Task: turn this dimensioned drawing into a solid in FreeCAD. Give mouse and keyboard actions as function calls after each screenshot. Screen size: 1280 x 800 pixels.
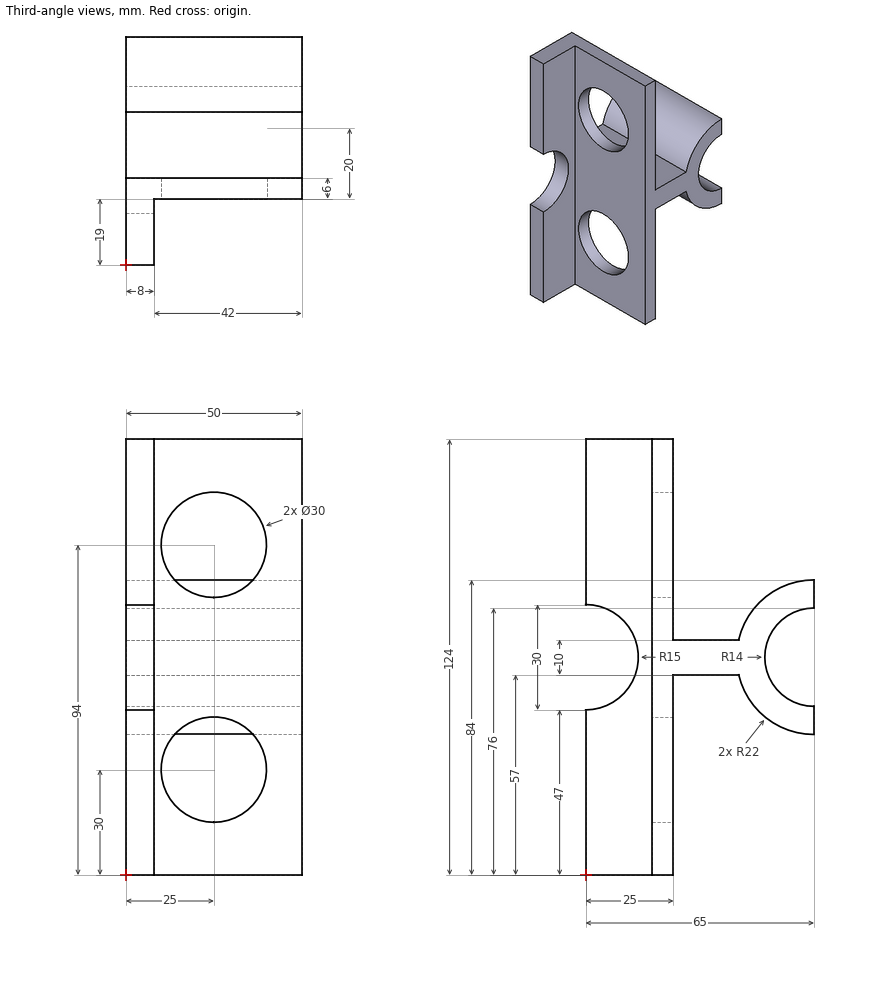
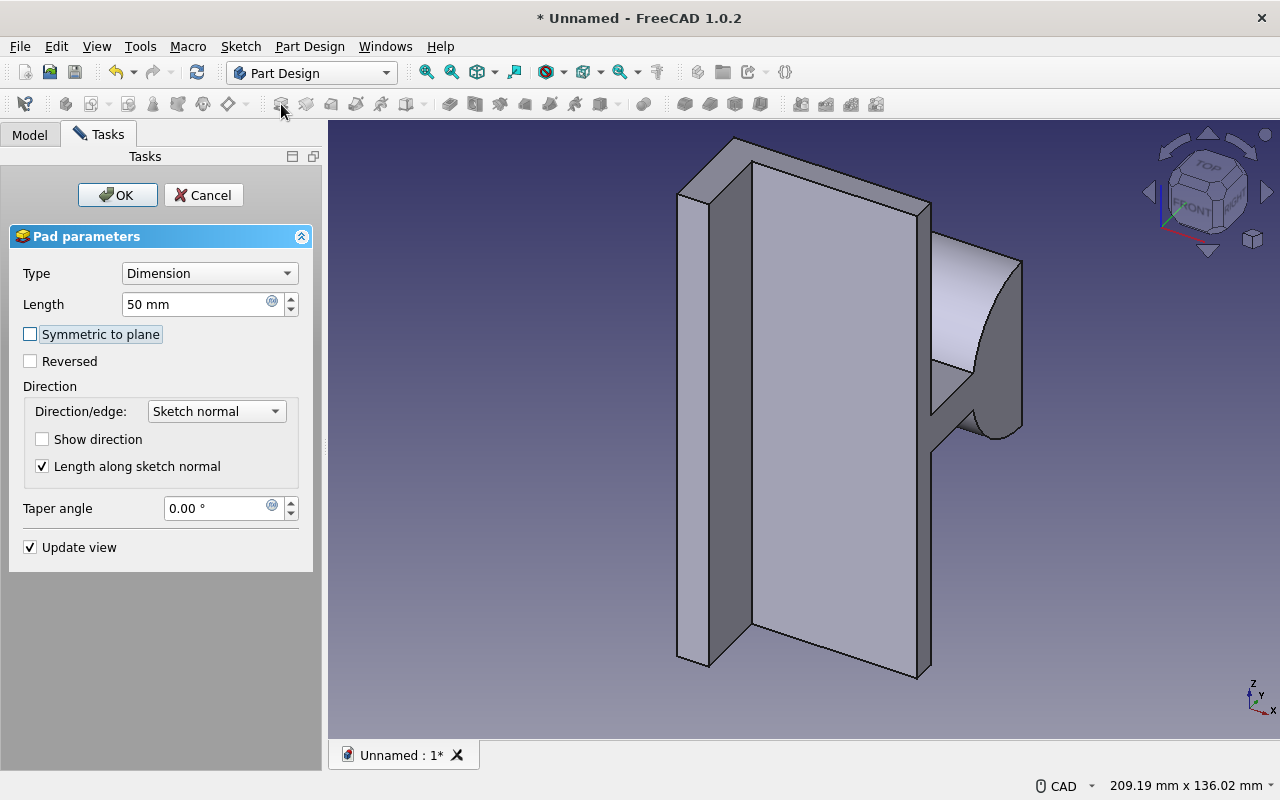
click(118, 195)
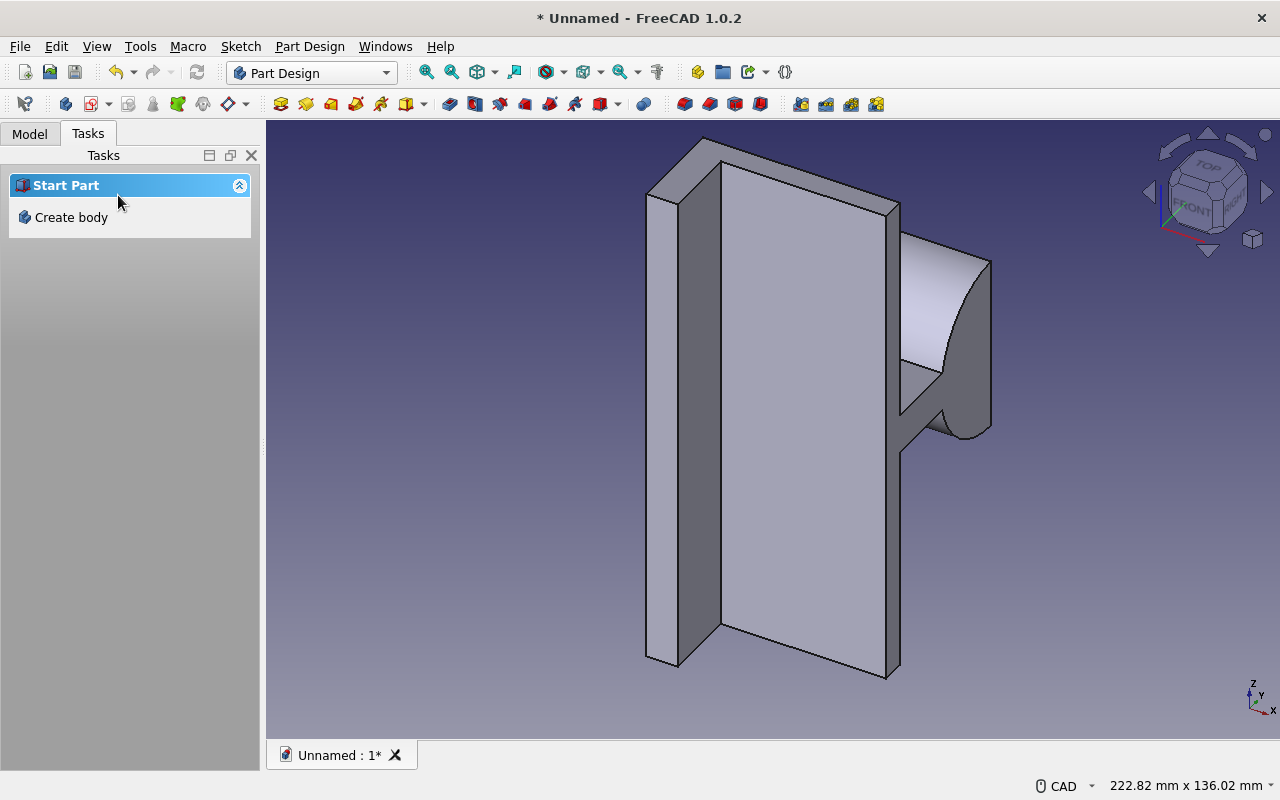
key(v)
key(f)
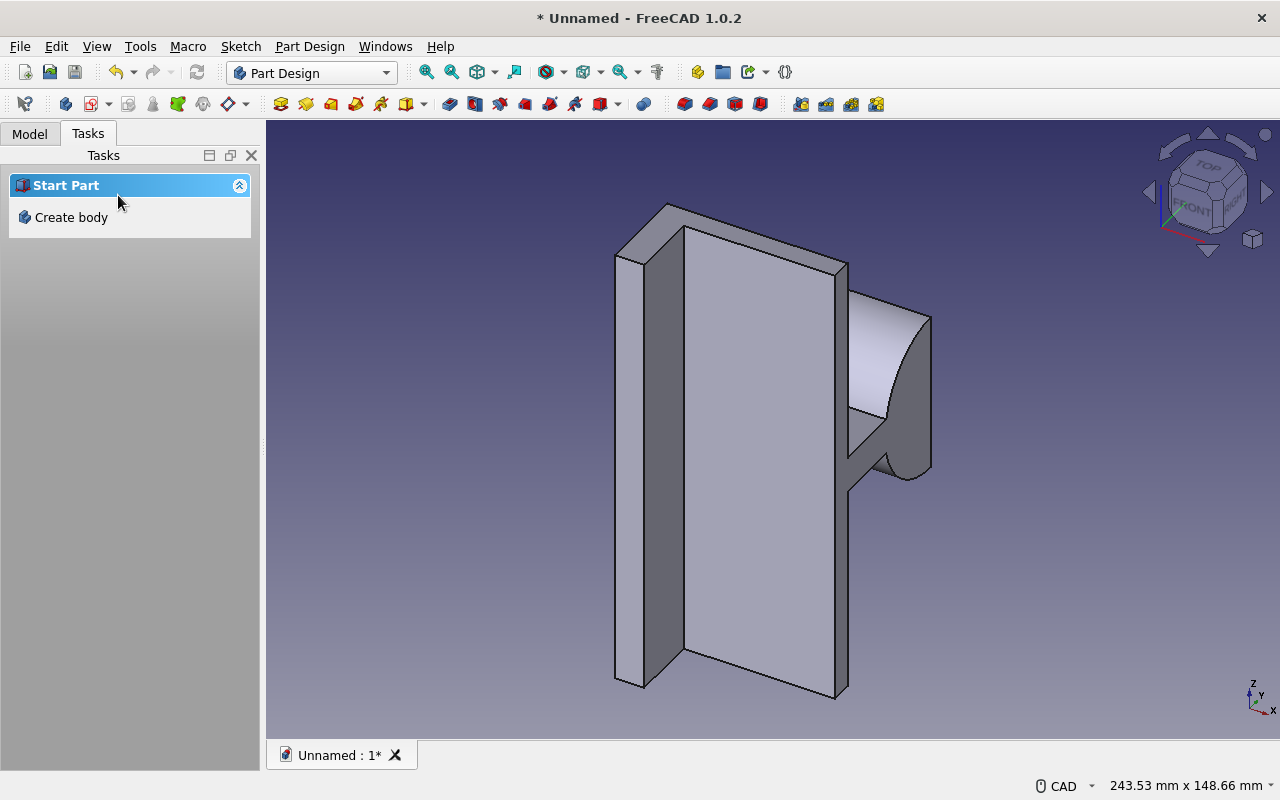
click(90, 104)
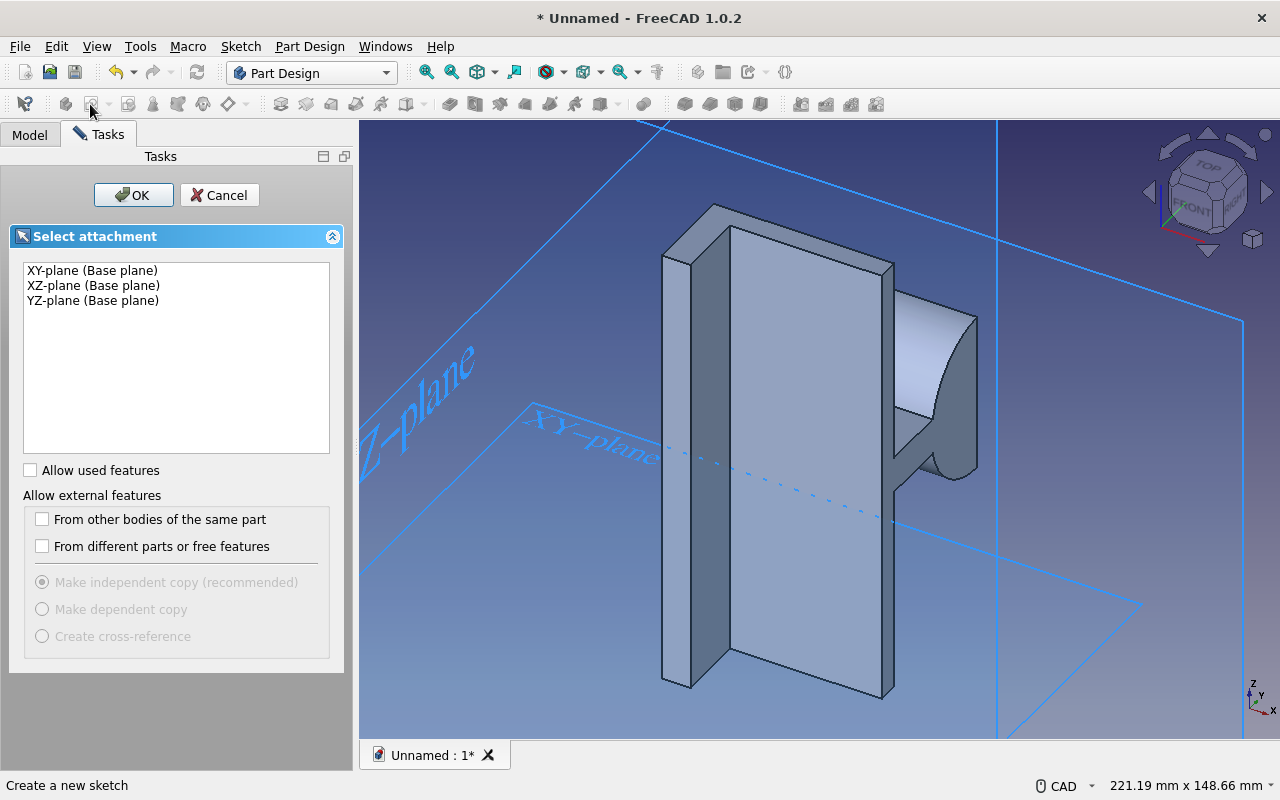
click(84, 300)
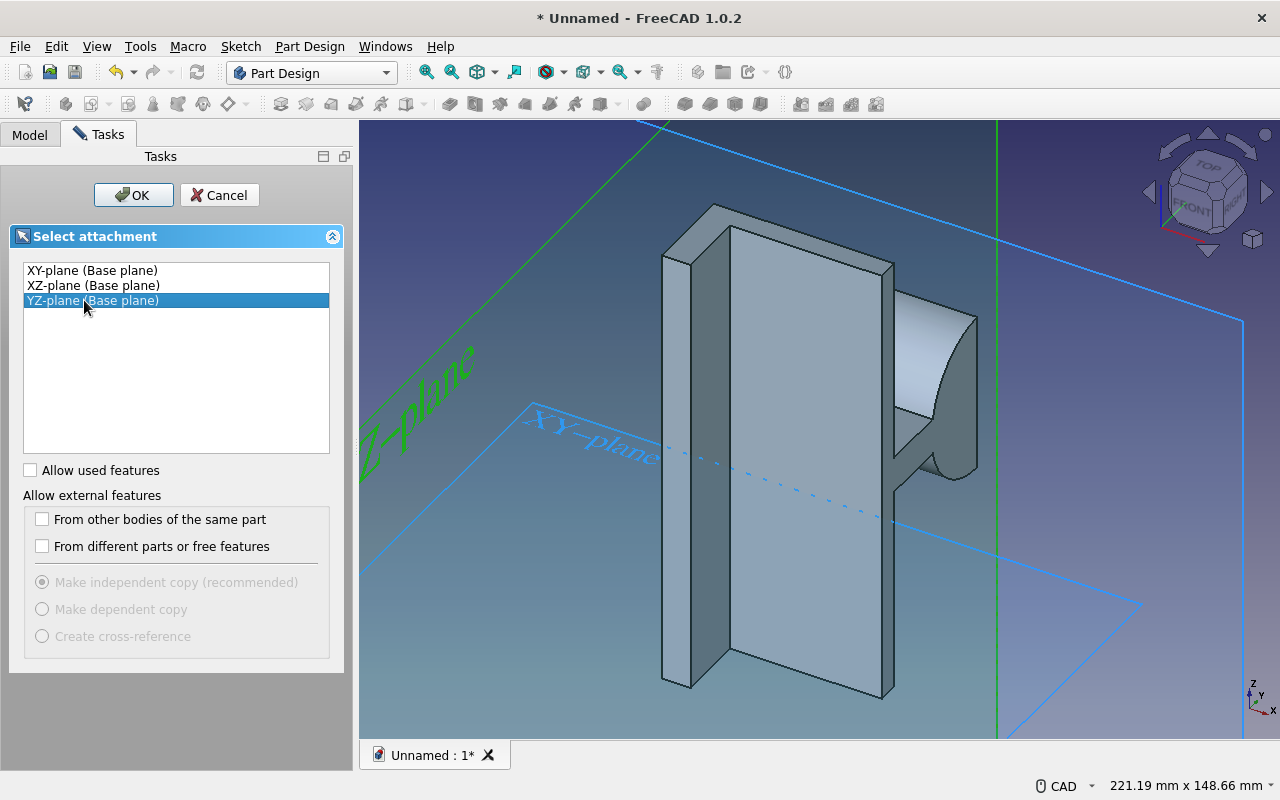
click(134, 195)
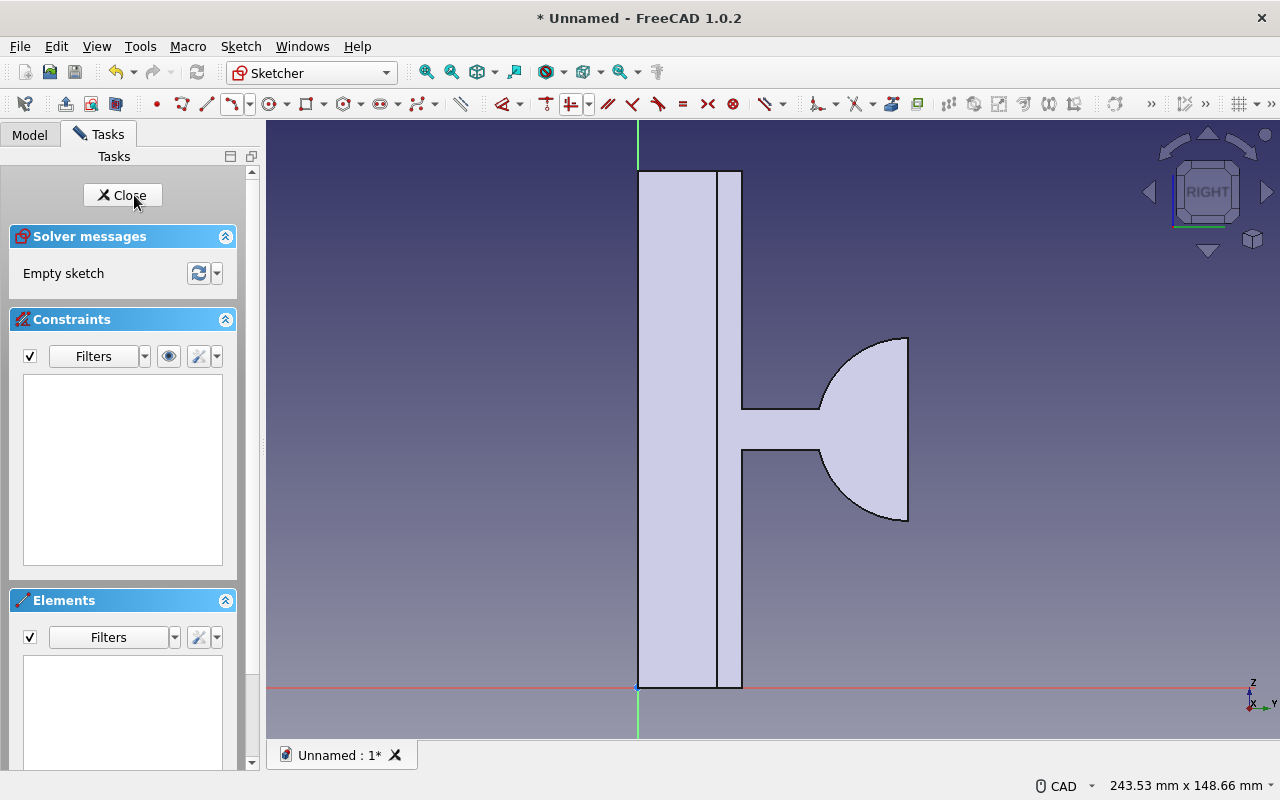
key(q)
key(s)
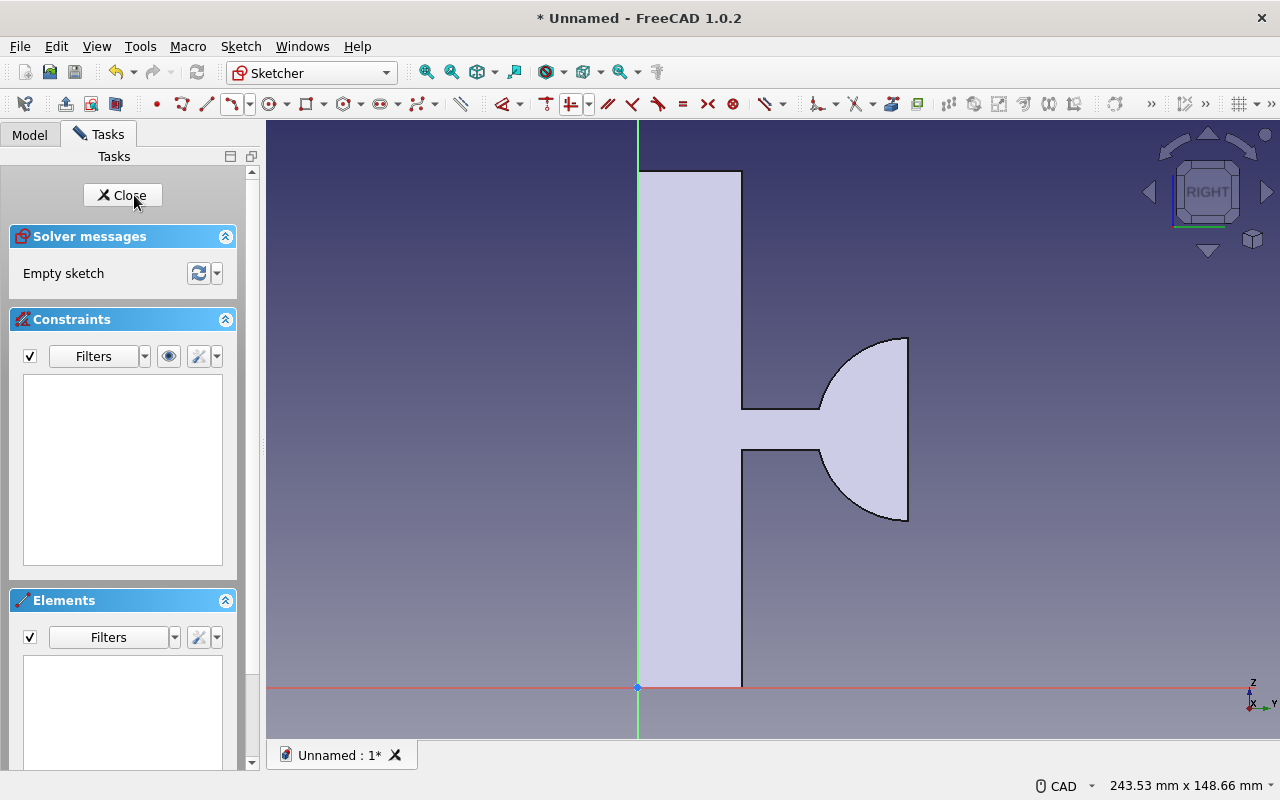
scroll(954, 430, up, 6)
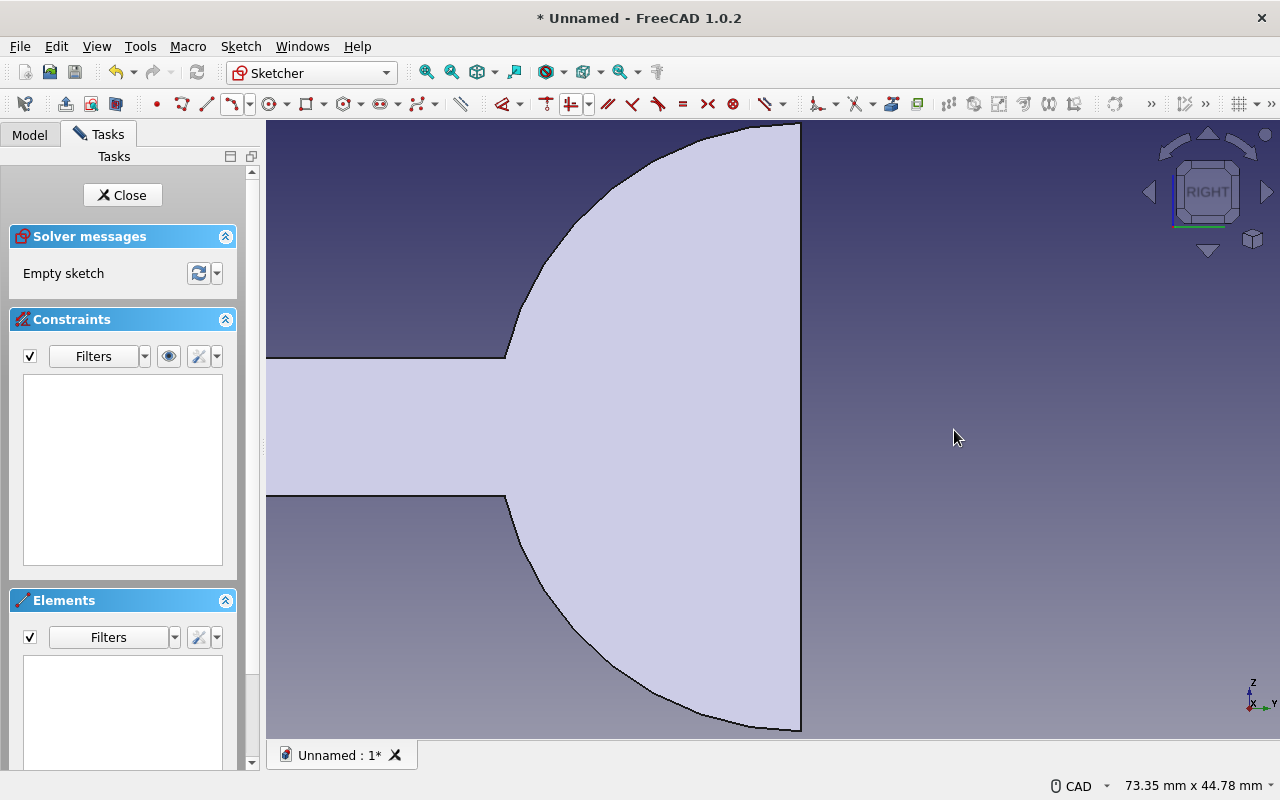
key(g)
key(l)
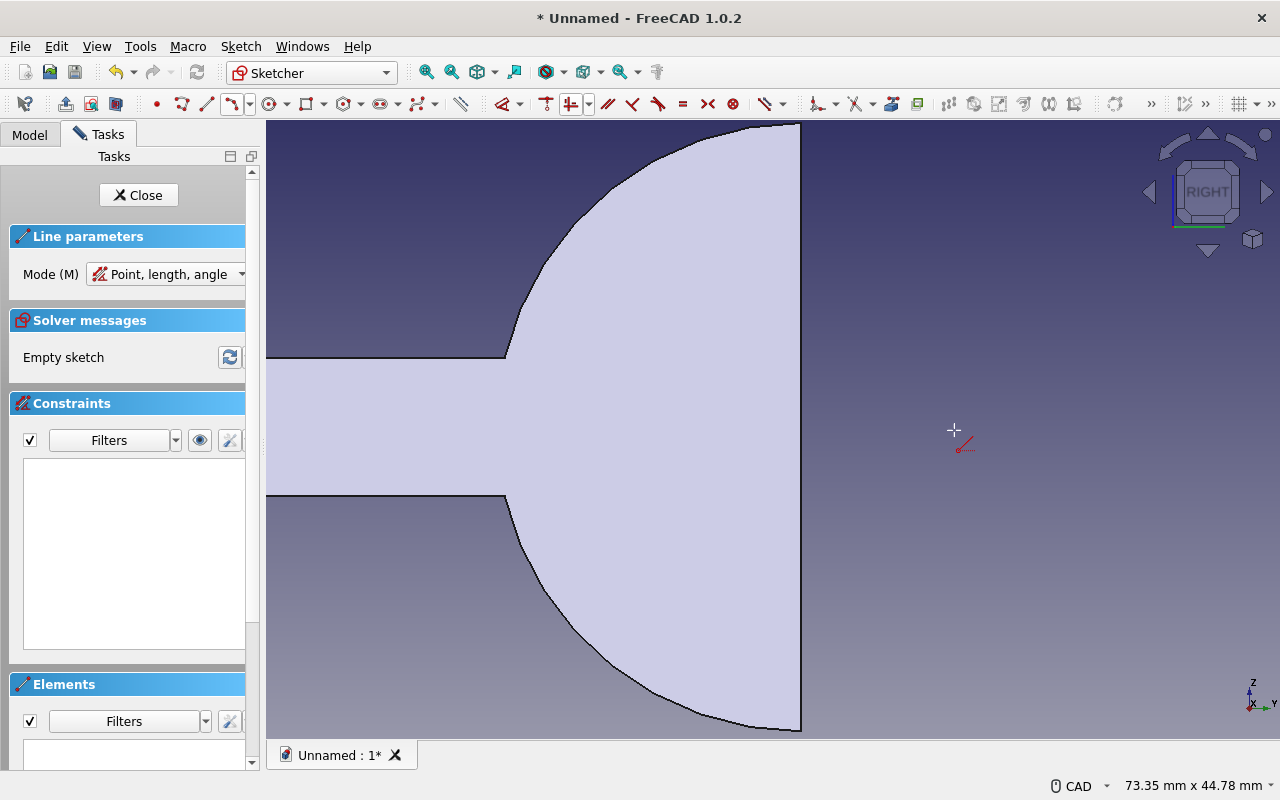
click(801, 234)
click(801, 621)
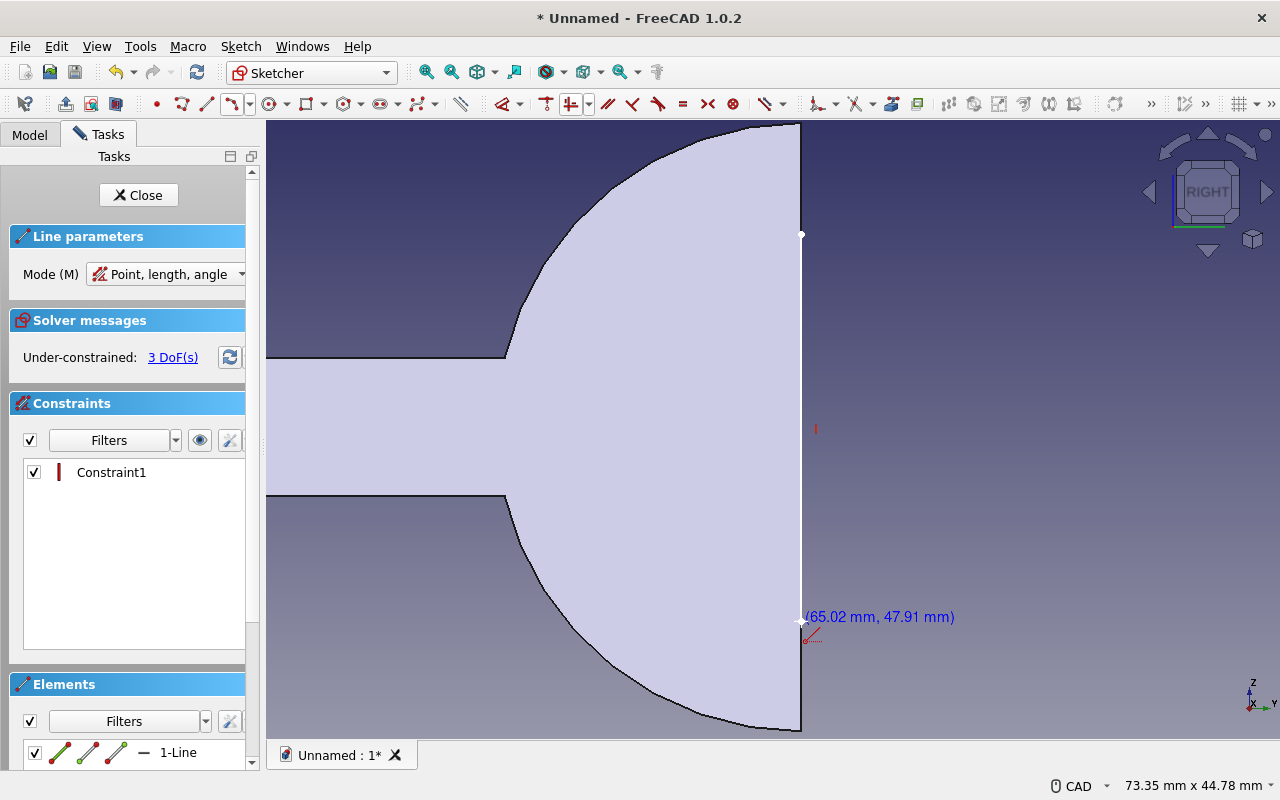
click(232, 104)